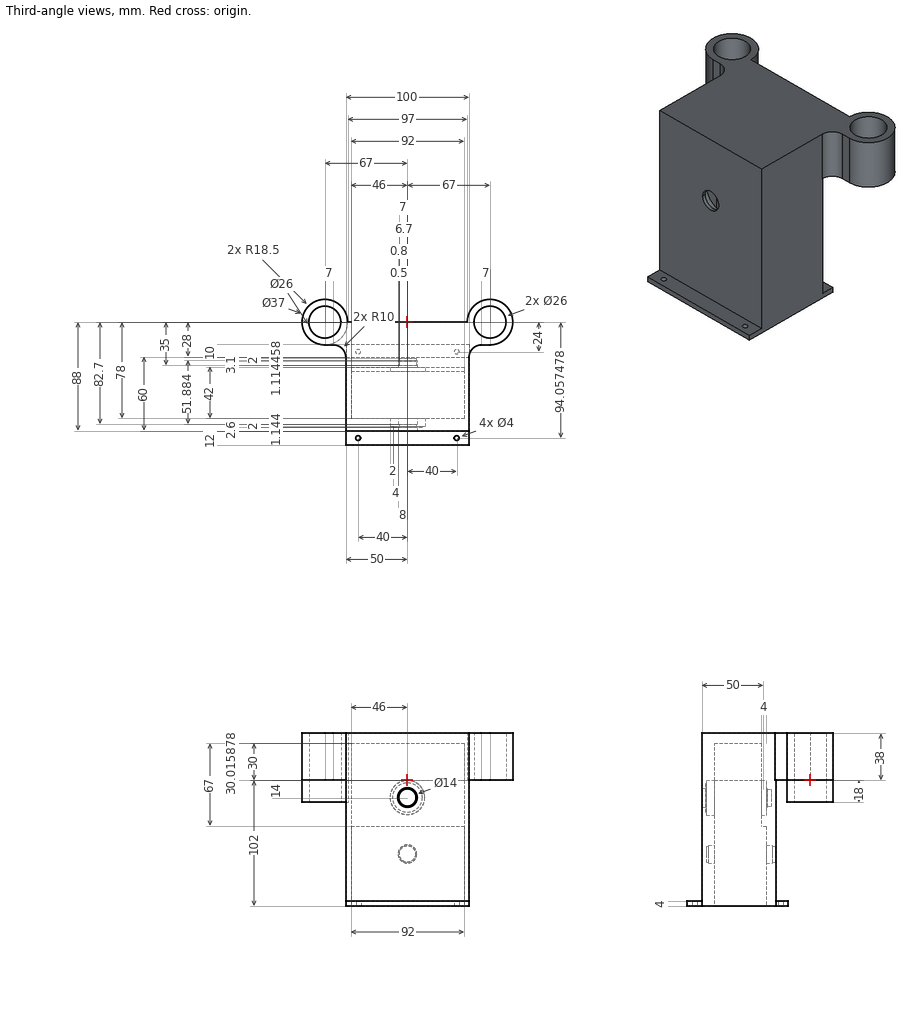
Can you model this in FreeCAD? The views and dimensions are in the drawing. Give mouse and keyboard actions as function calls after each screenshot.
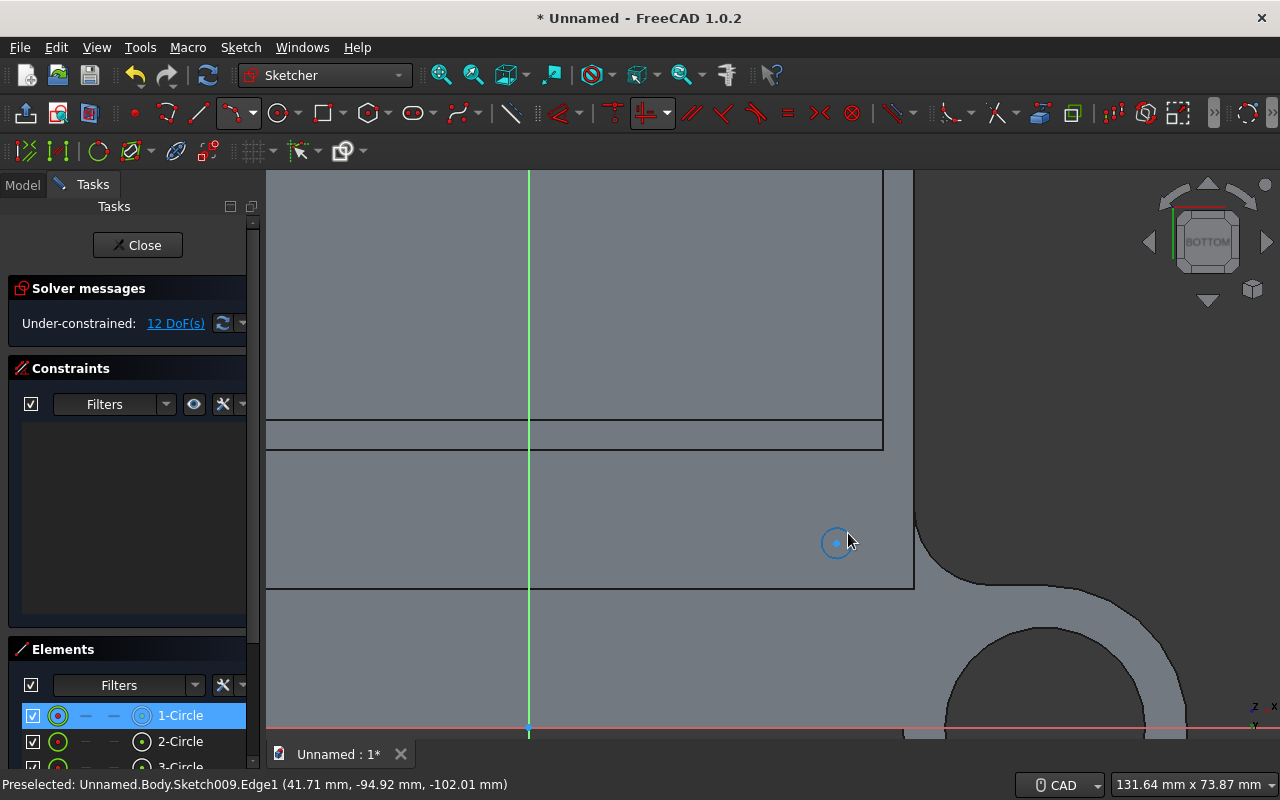
click(848, 533)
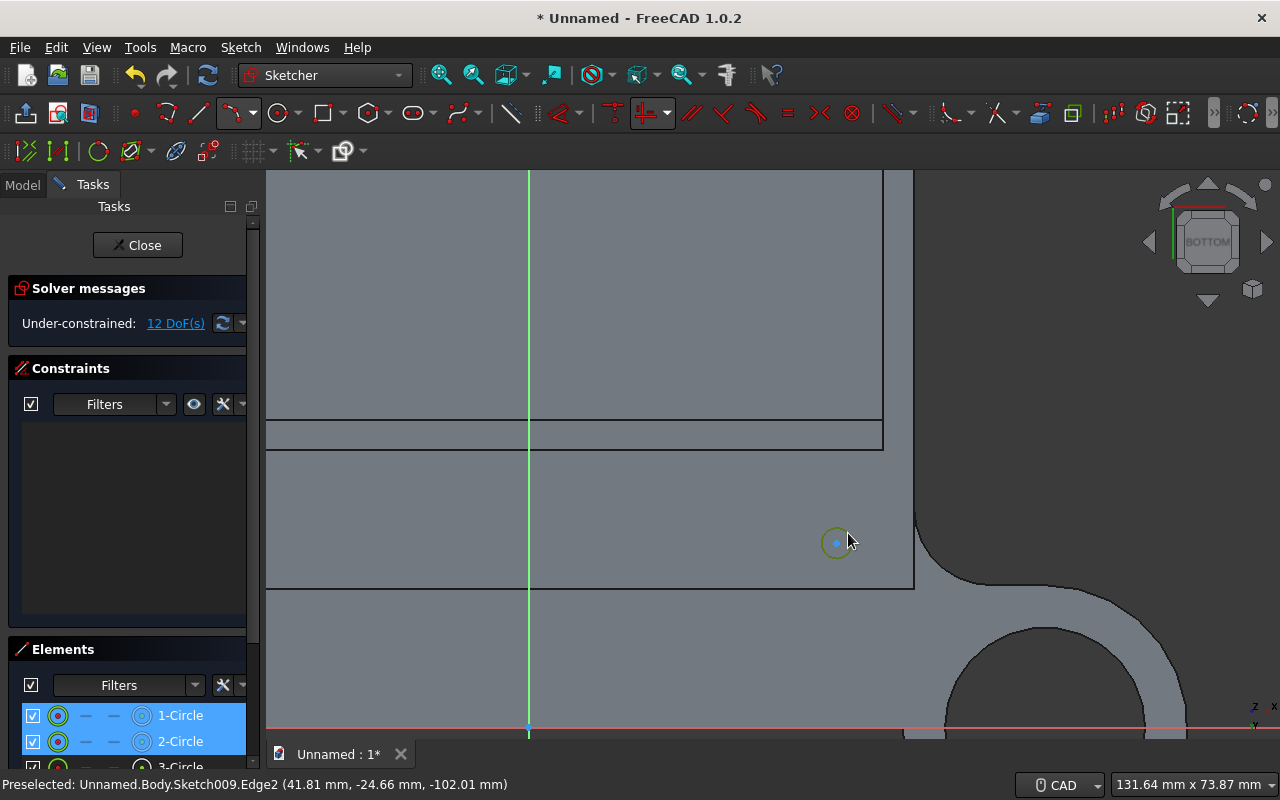
scroll(848, 533, down, 4)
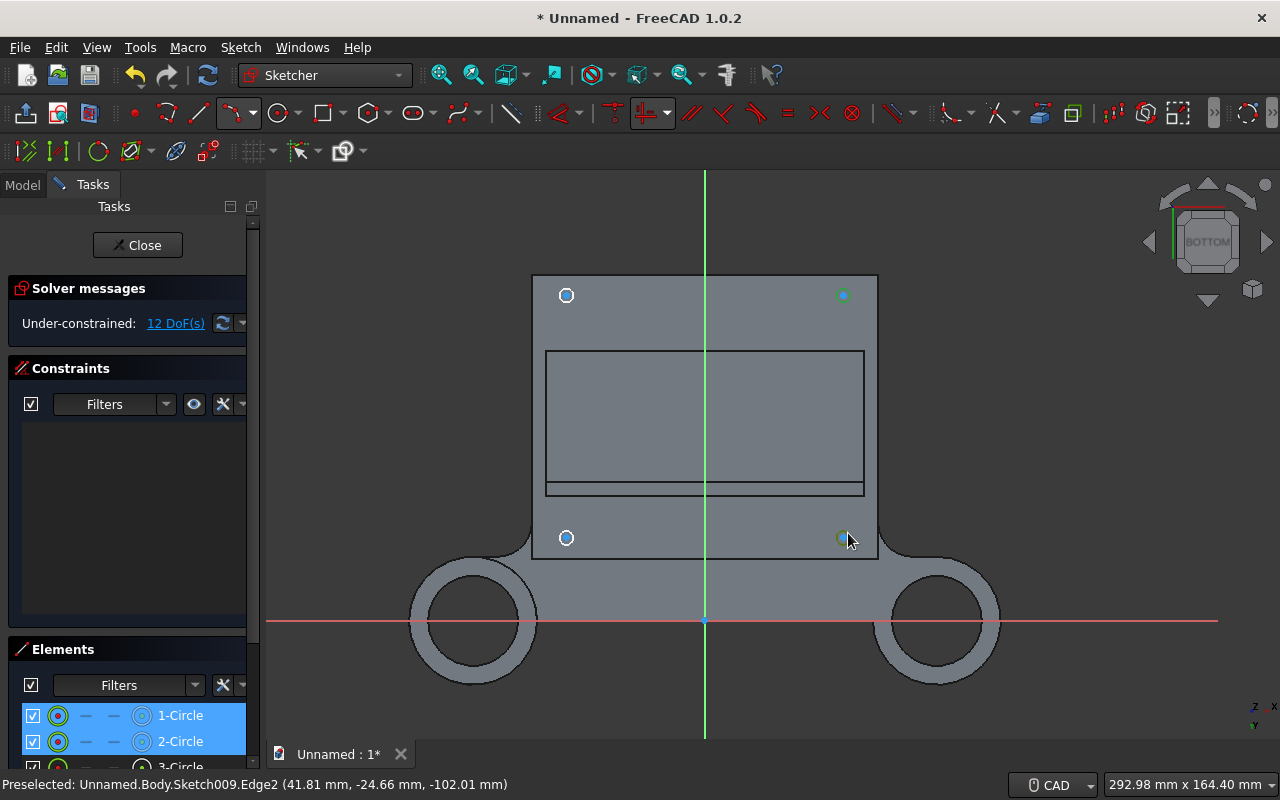
scroll(571, 291, up, 4)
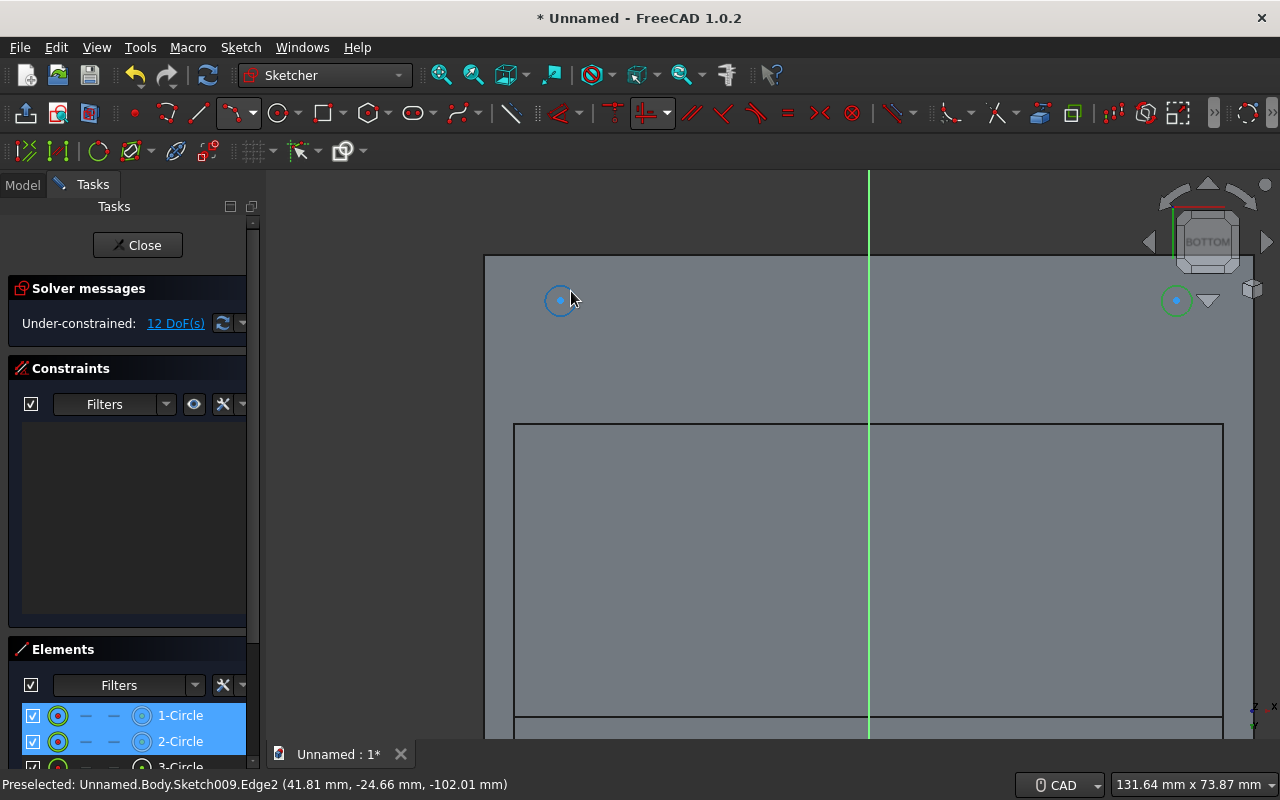
click(571, 290)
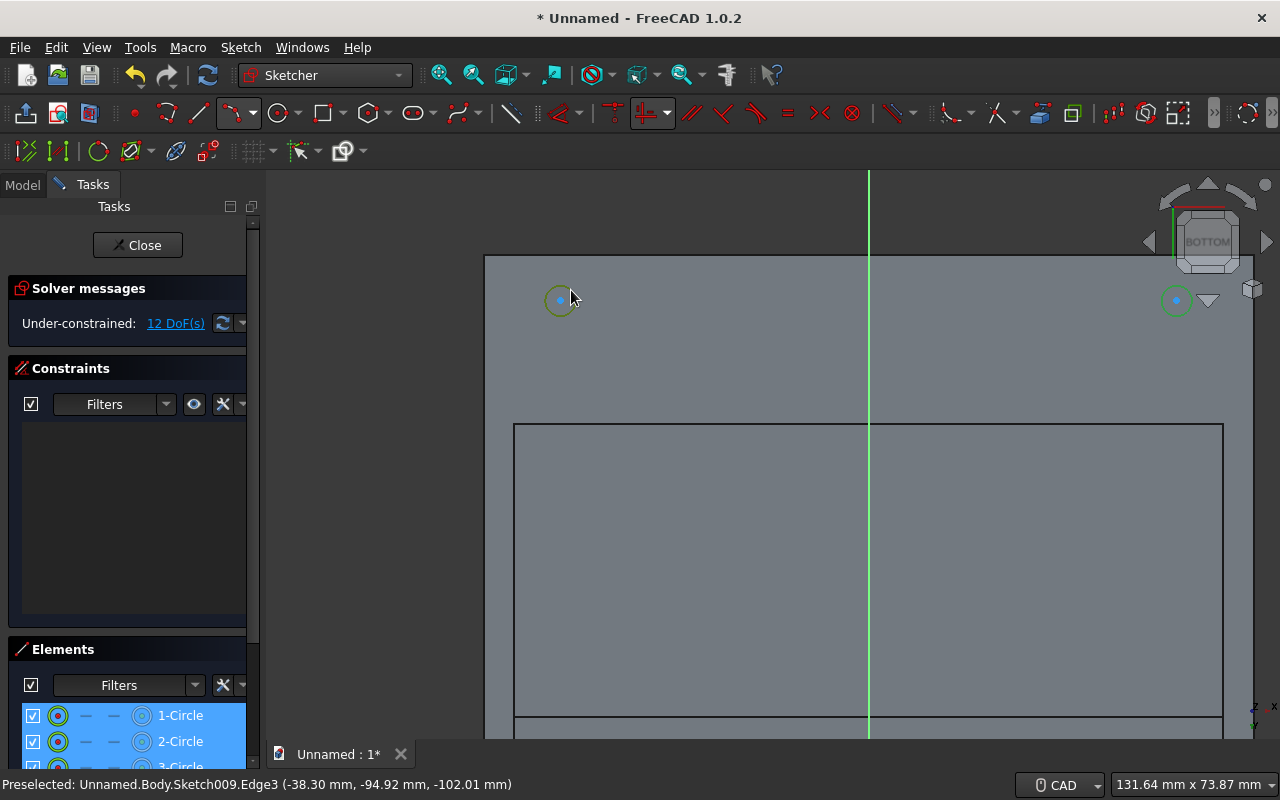
scroll(570, 291, down, 4)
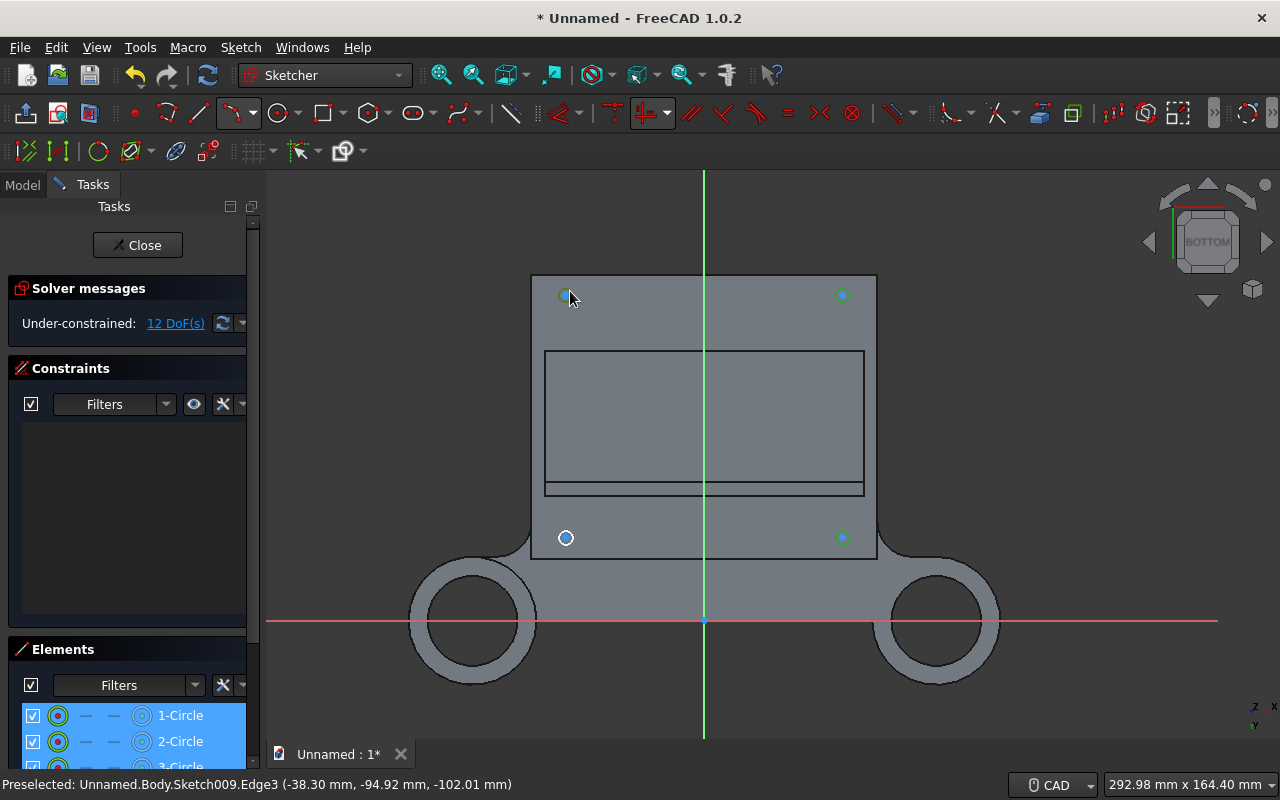
scroll(571, 533, up, 4)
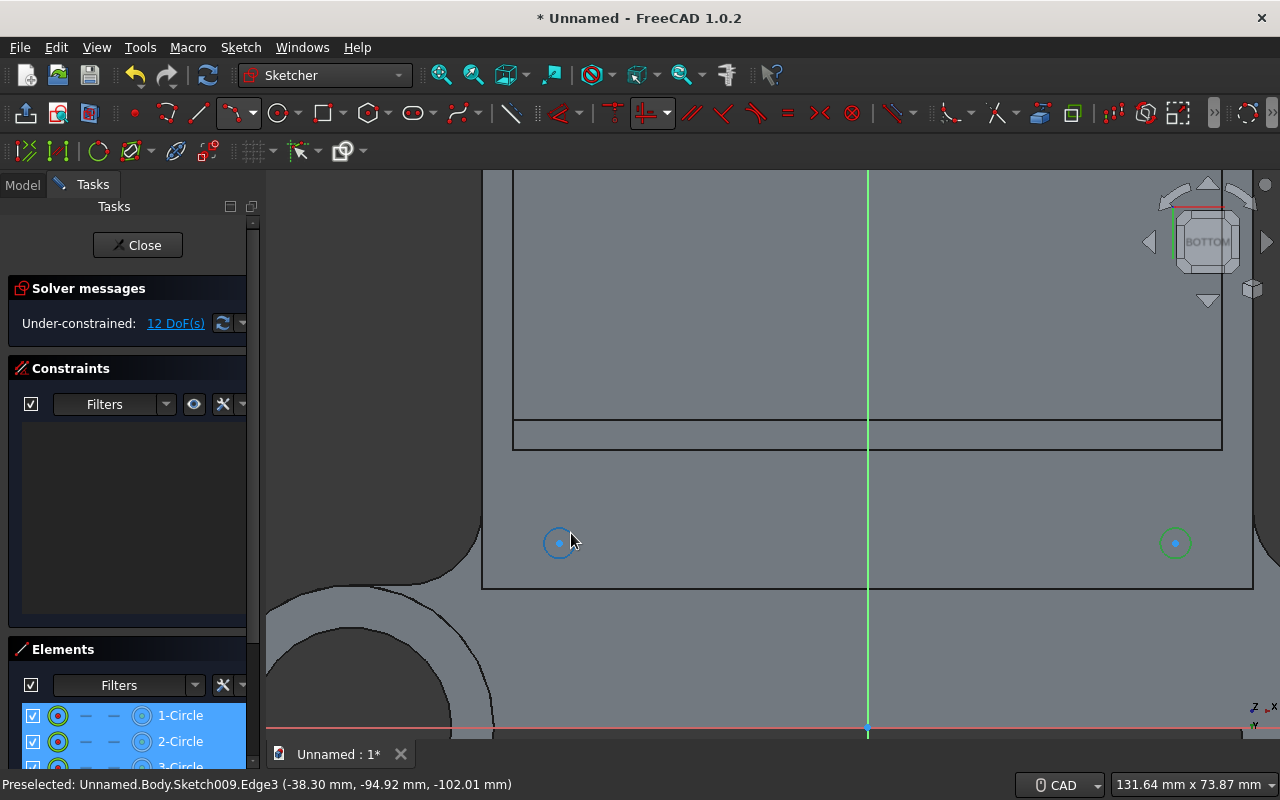
click(570, 533)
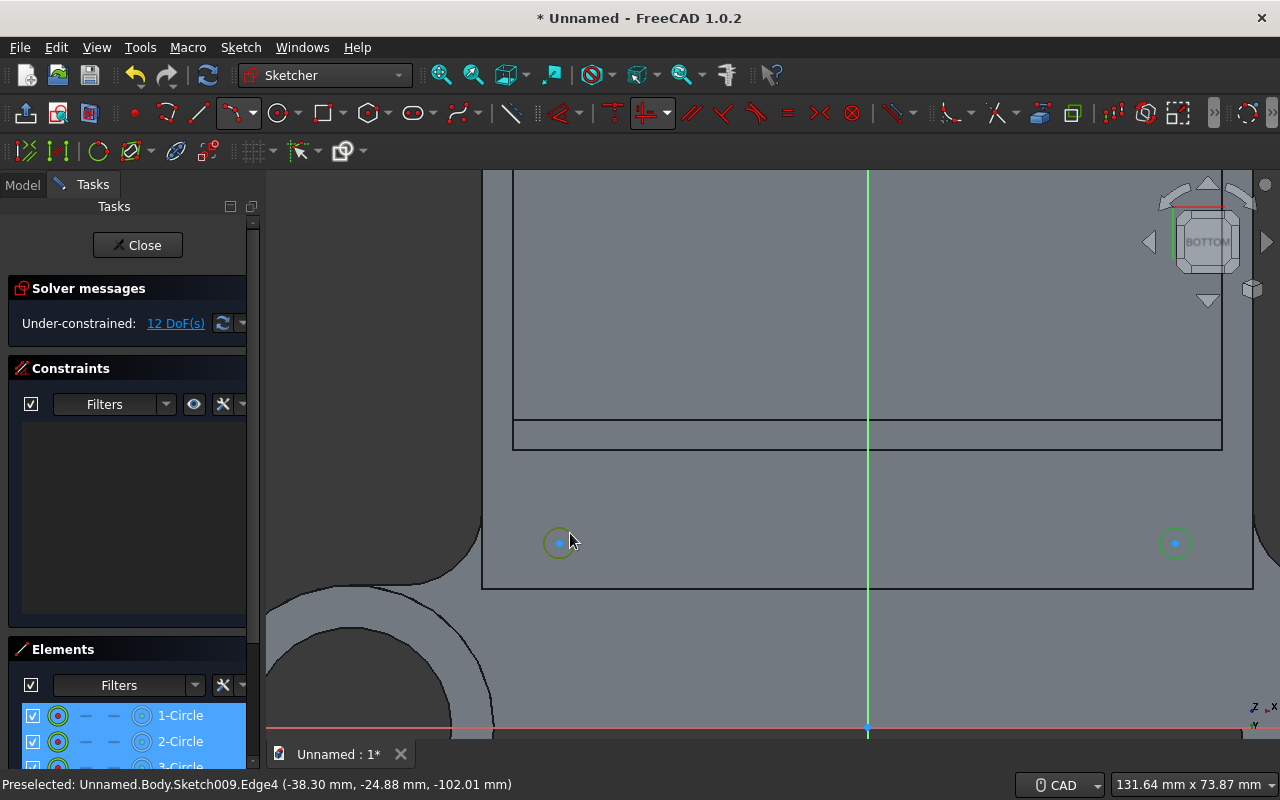
key(e)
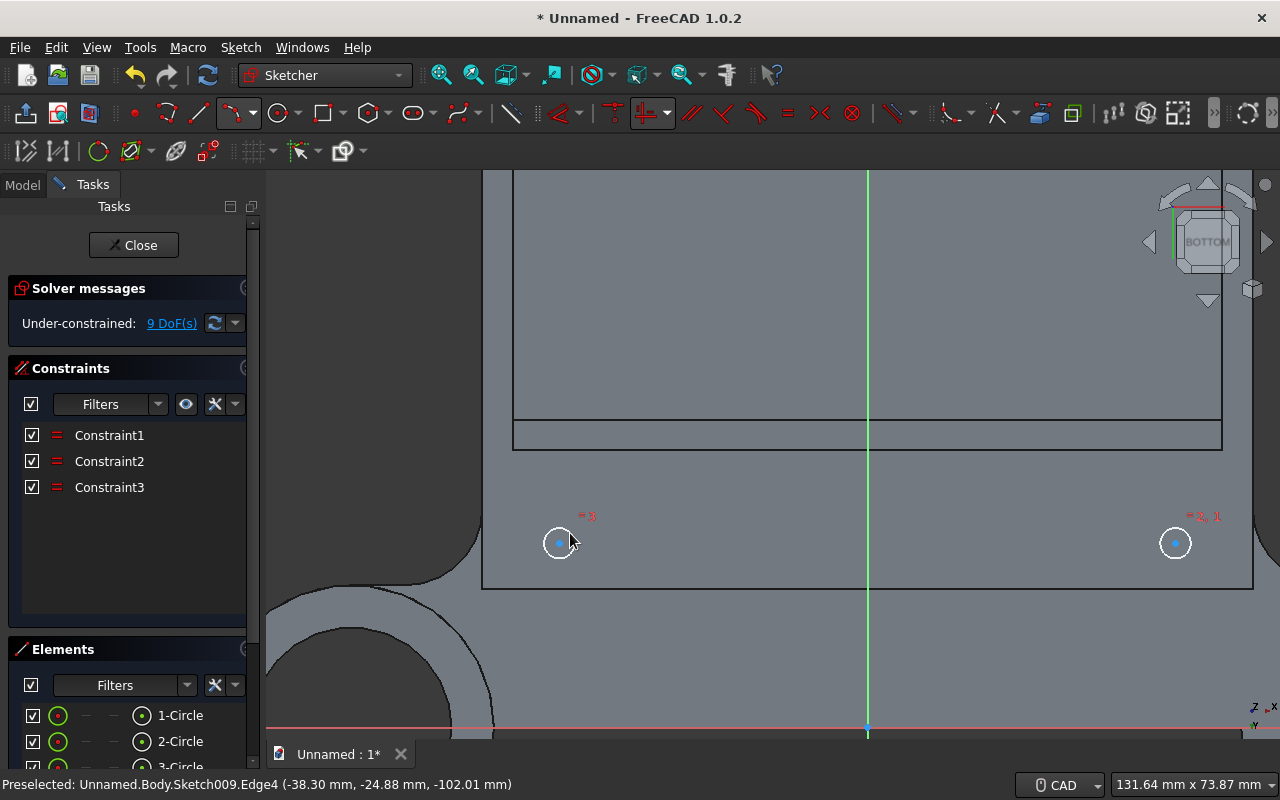
scroll(571, 533, down, 4)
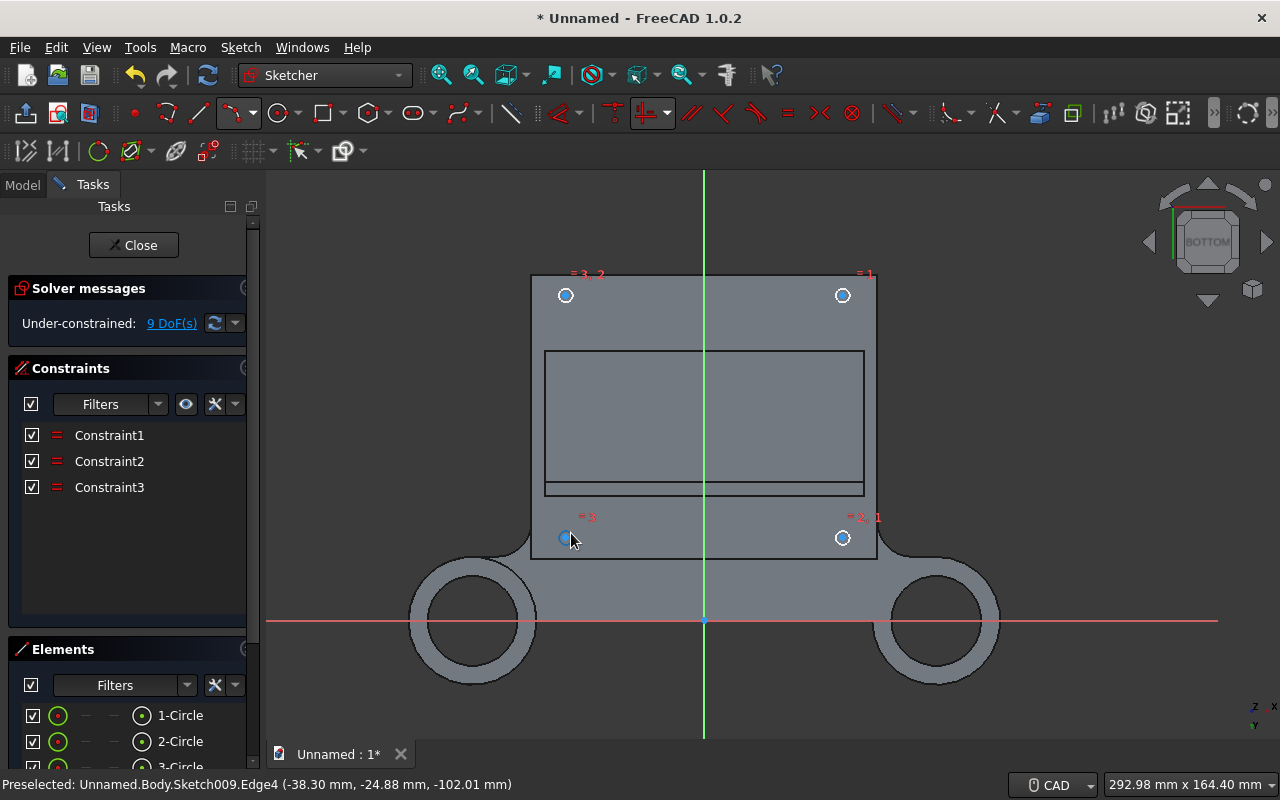
click(843, 296)